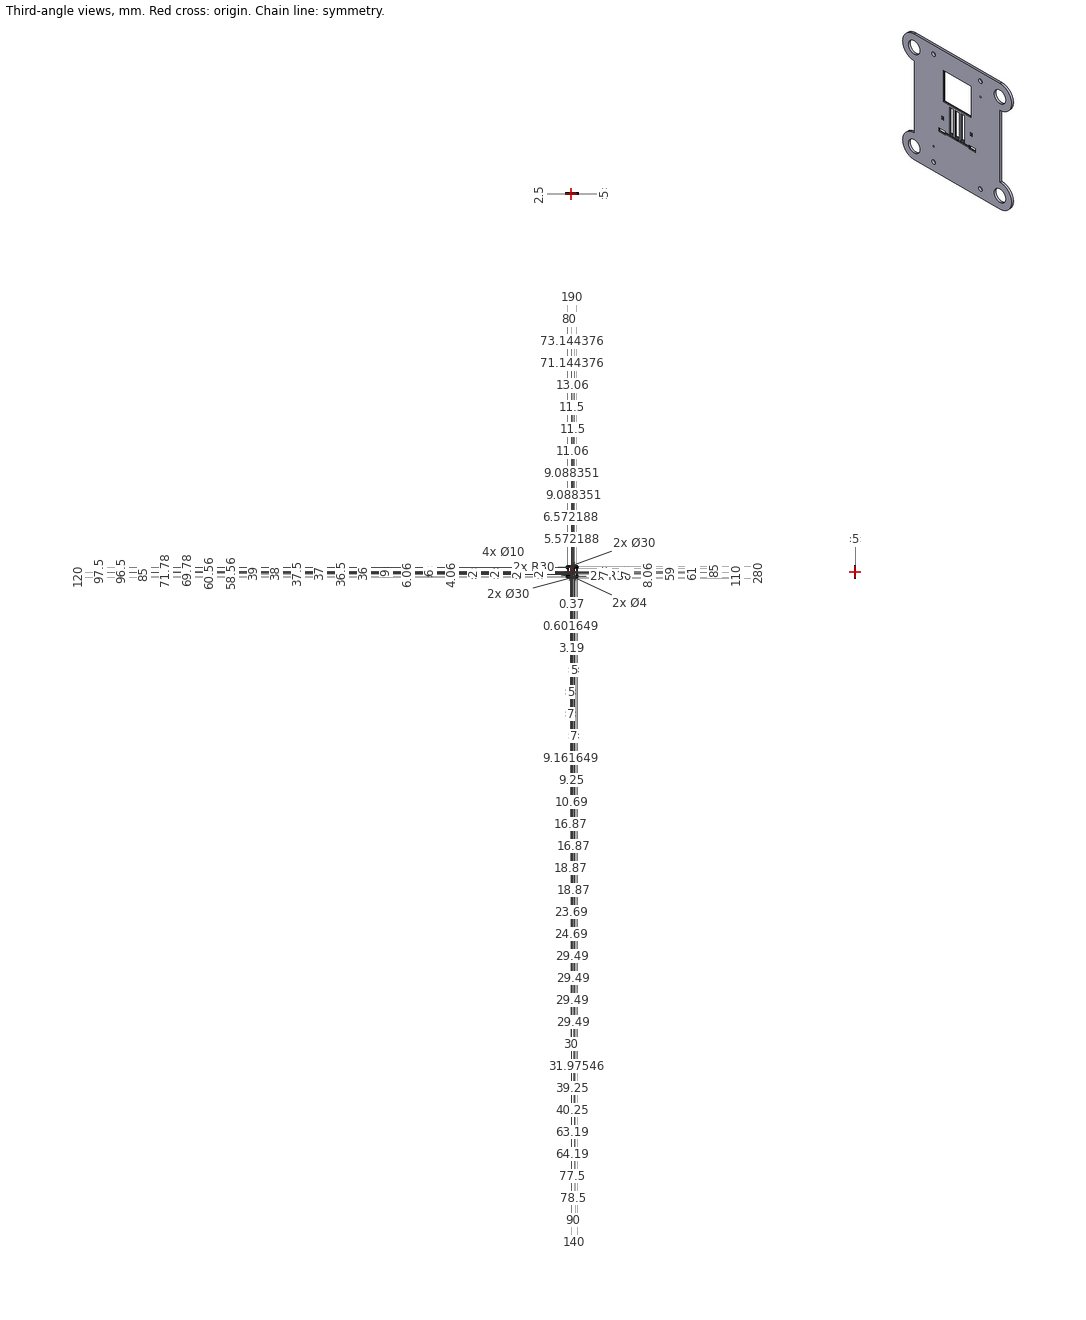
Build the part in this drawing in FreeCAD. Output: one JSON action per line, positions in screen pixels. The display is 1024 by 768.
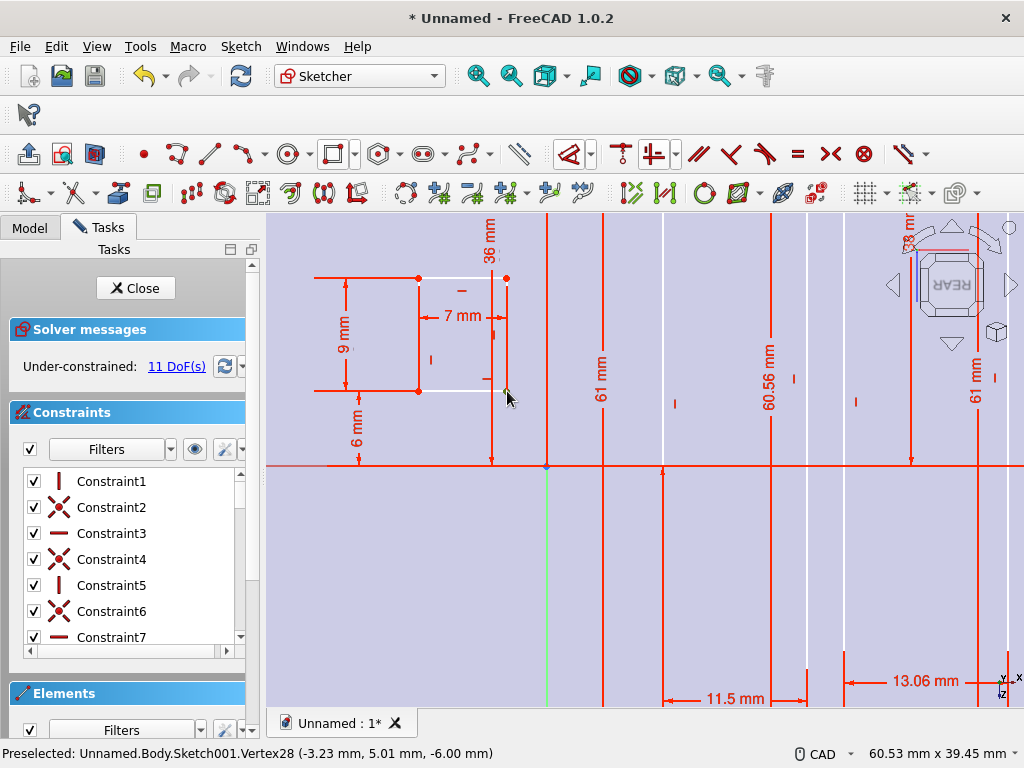
{"action": "left_click", "coordinate": [590, 154]}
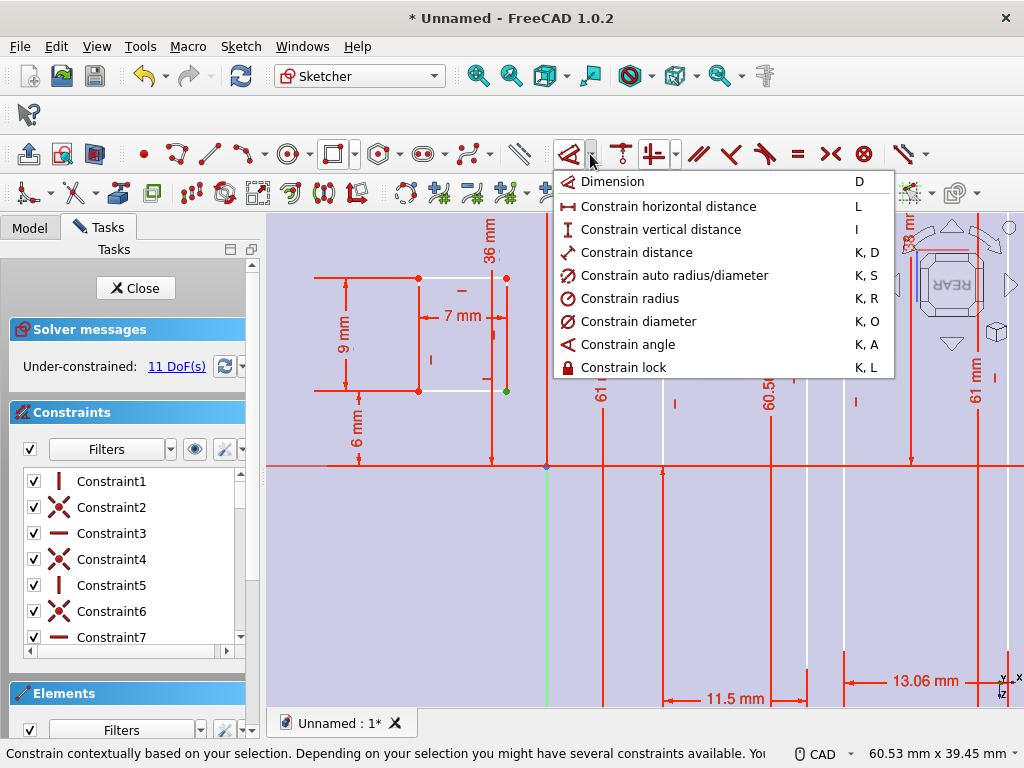
{"action": "left_click", "coordinate": [724, 206]}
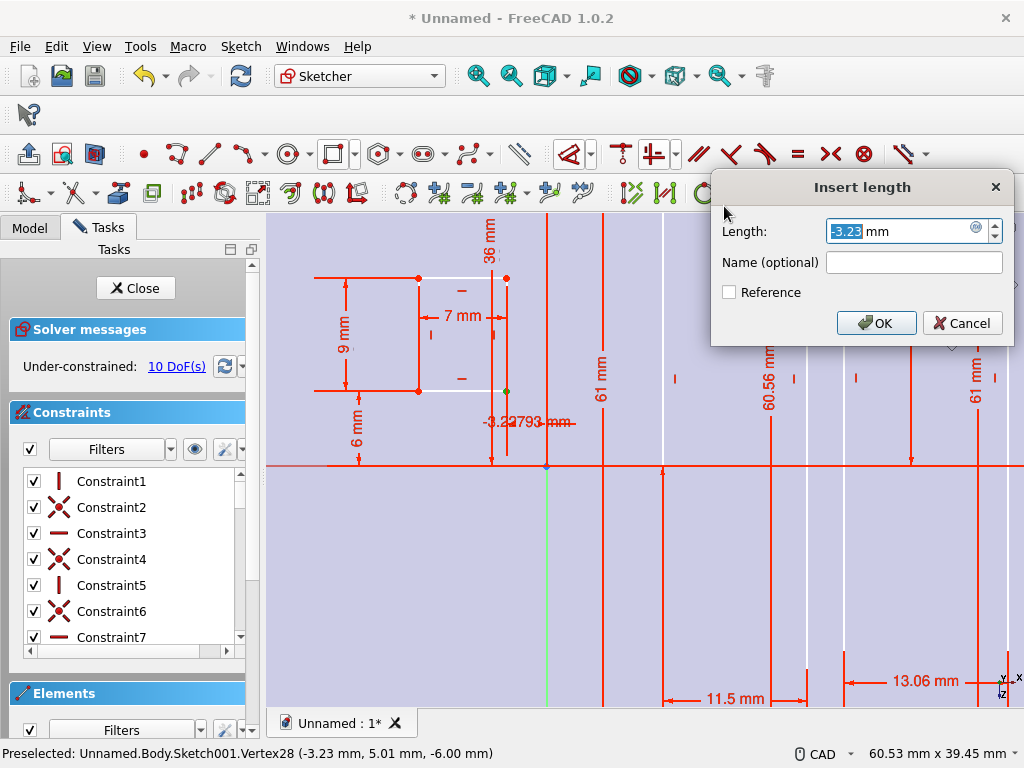
{"action": "type", "text": "-3.19"}
{"action": "key", "text": "Return"}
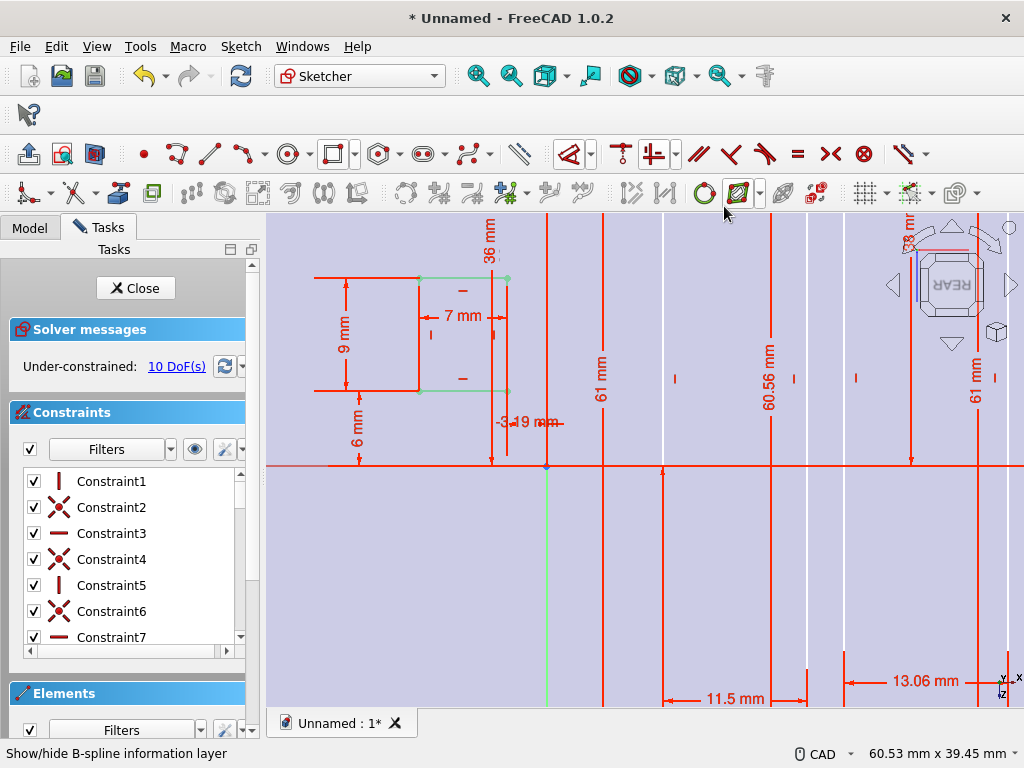
{"action": "scroll", "coordinate": [508, 395], "scroll_direction": "down", "scroll_amount": 9}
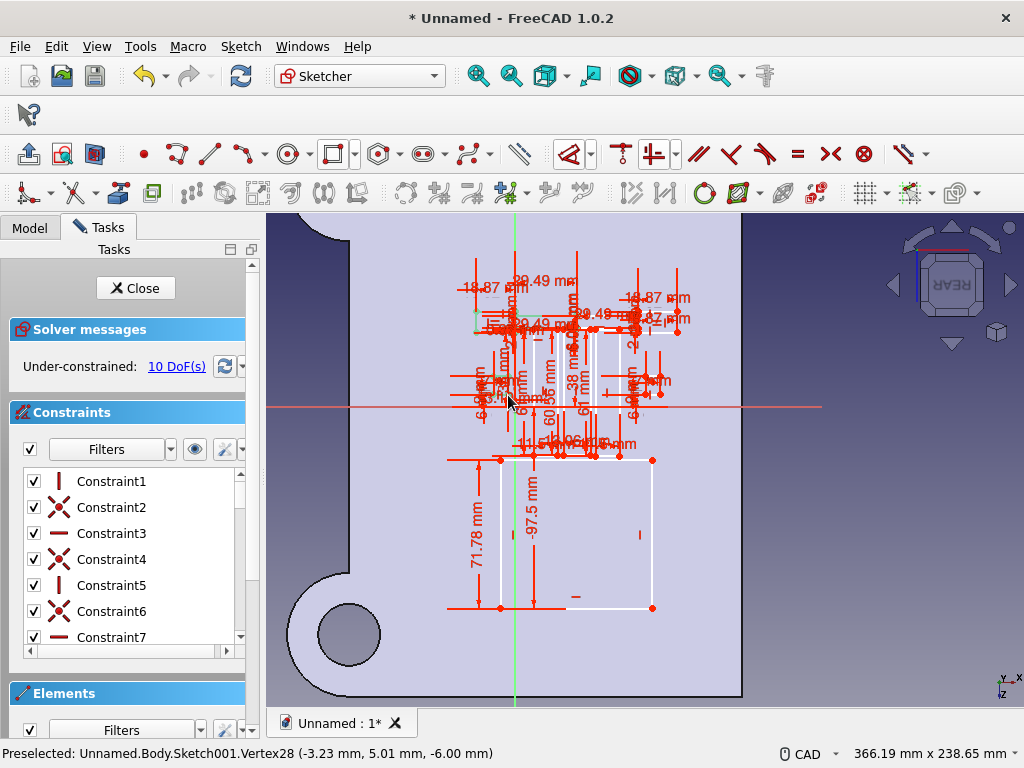
{"action": "scroll", "coordinate": [596, 330], "scroll_direction": "up", "scroll_amount": 5}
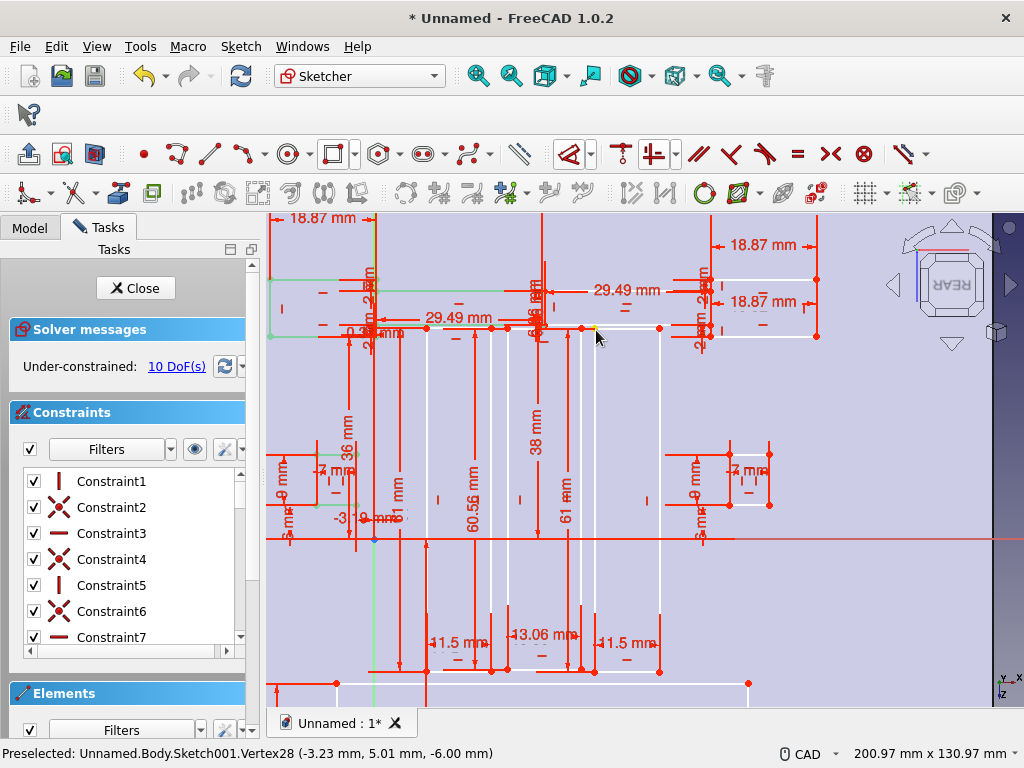
{"action": "left_click", "coordinate": [595, 329]}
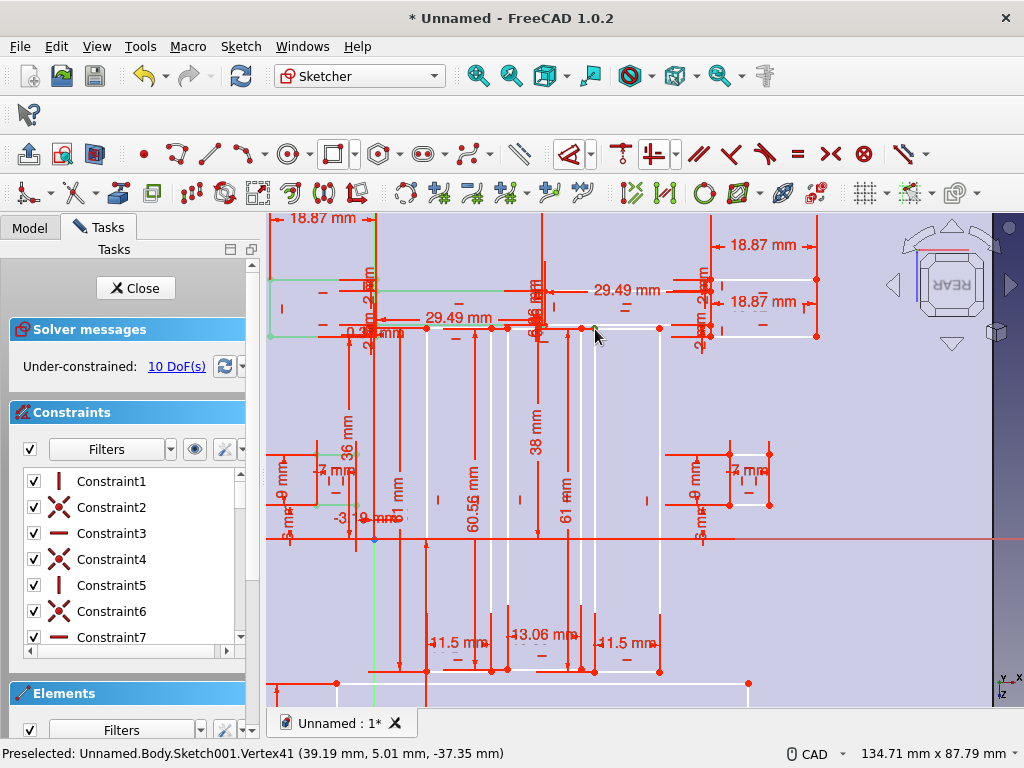
{"action": "key", "text": "i"}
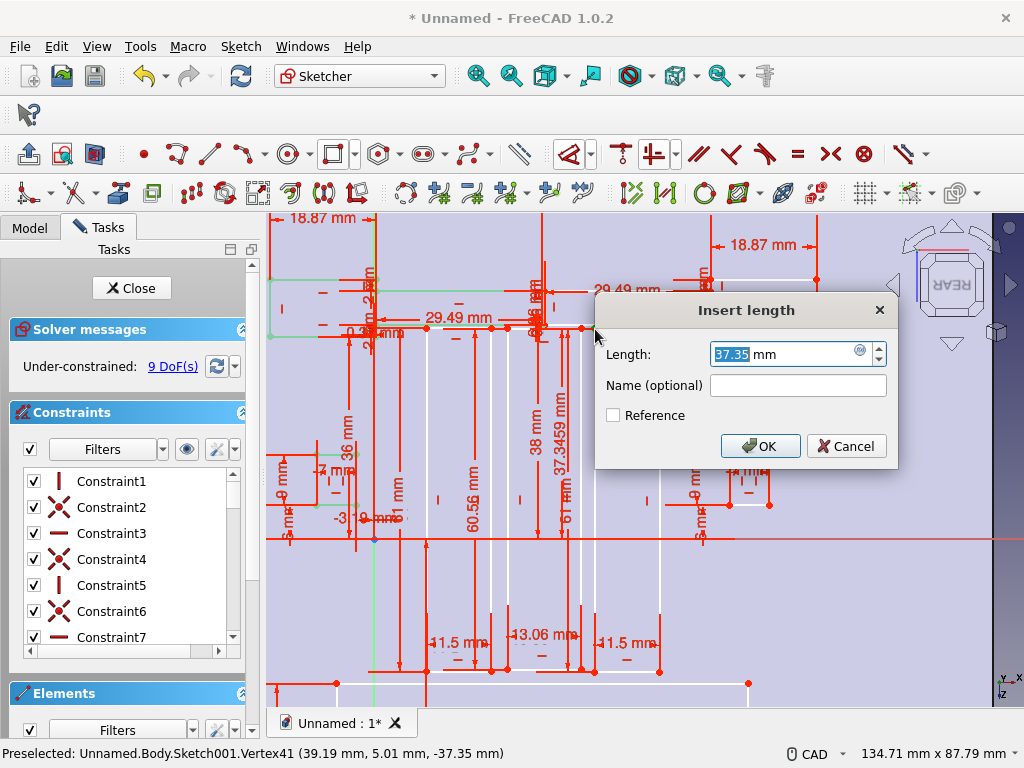
{"action": "type", "text": "37.5"}
{"action": "key", "text": "Return"}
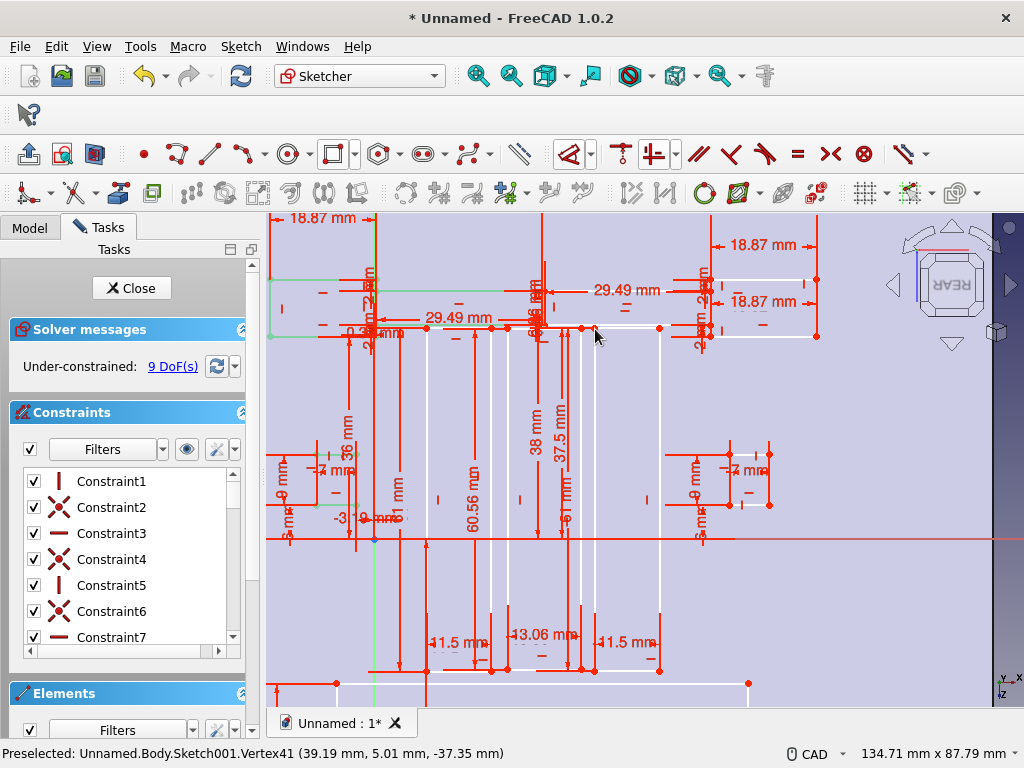
{"action": "left_click", "coordinate": [508, 329]}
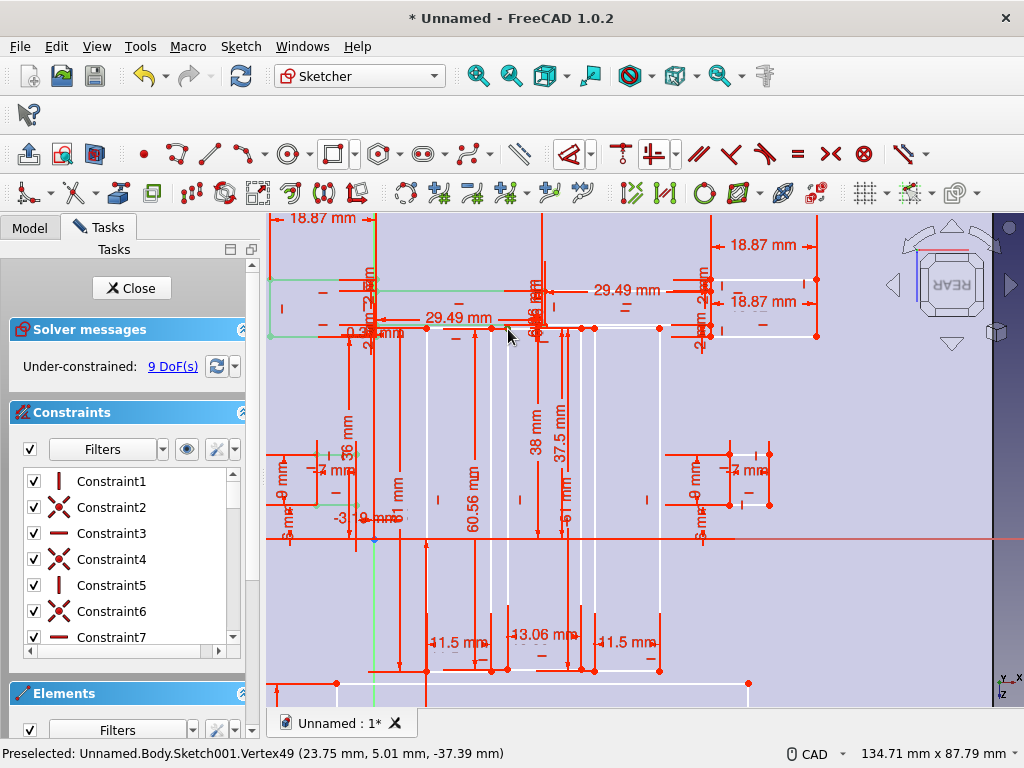
{"action": "key", "text": "i"}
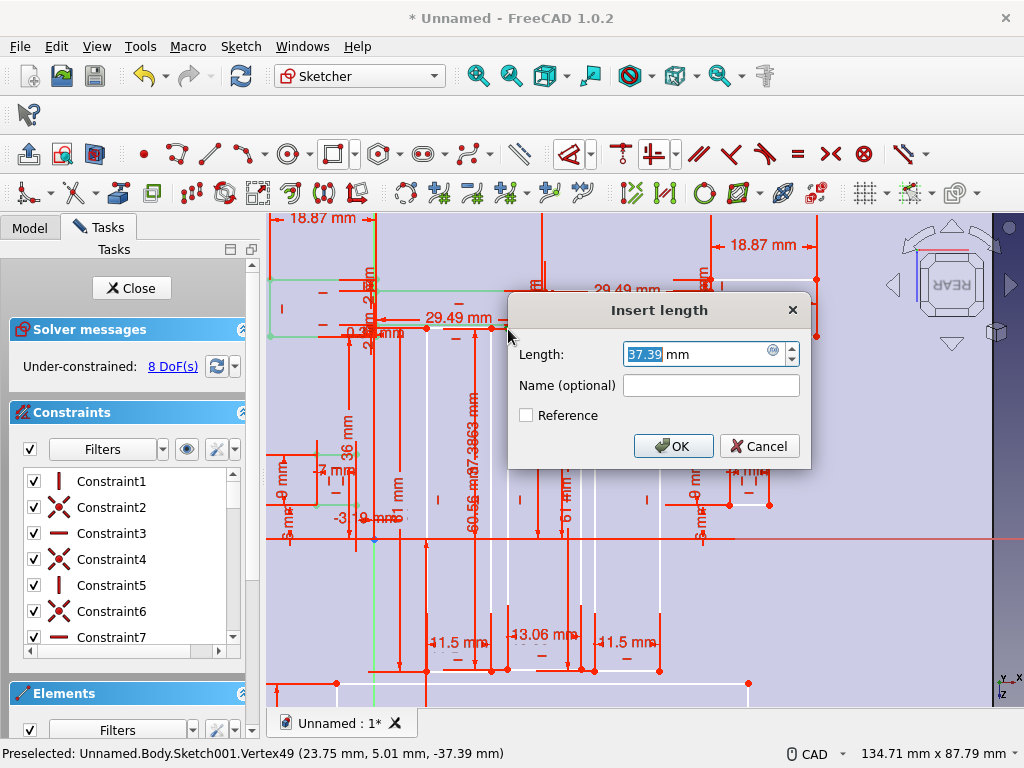
{"action": "type", "text": "37.5"}
{"action": "key", "text": "Return"}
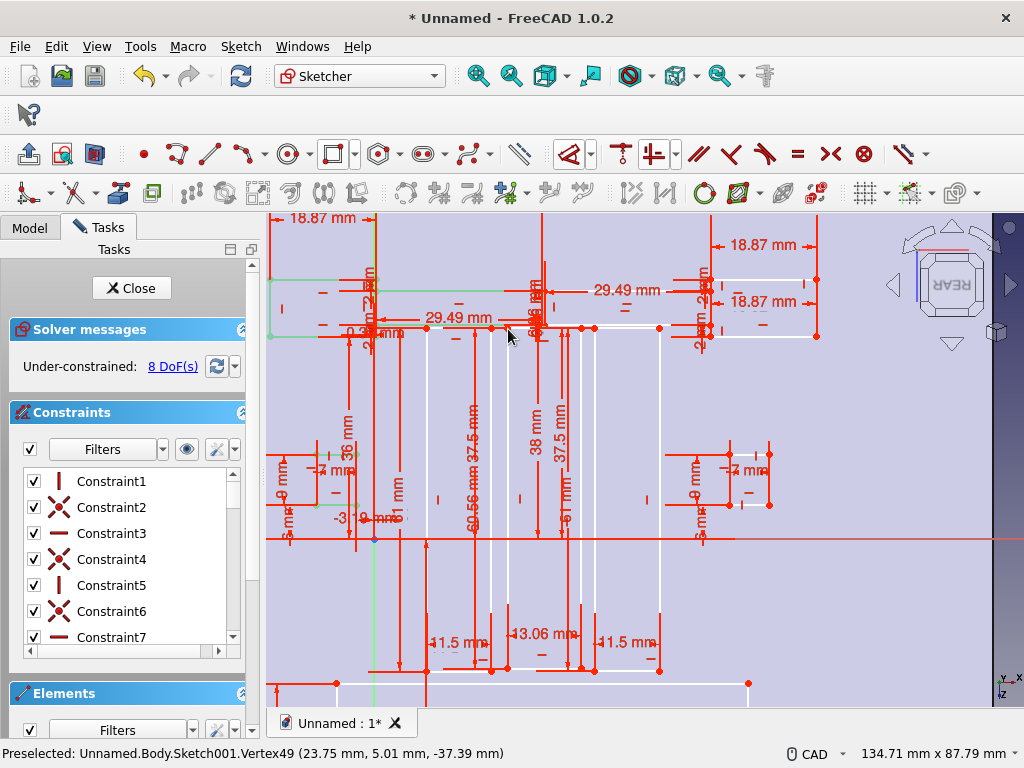
{"action": "left_click", "coordinate": [427, 328]}